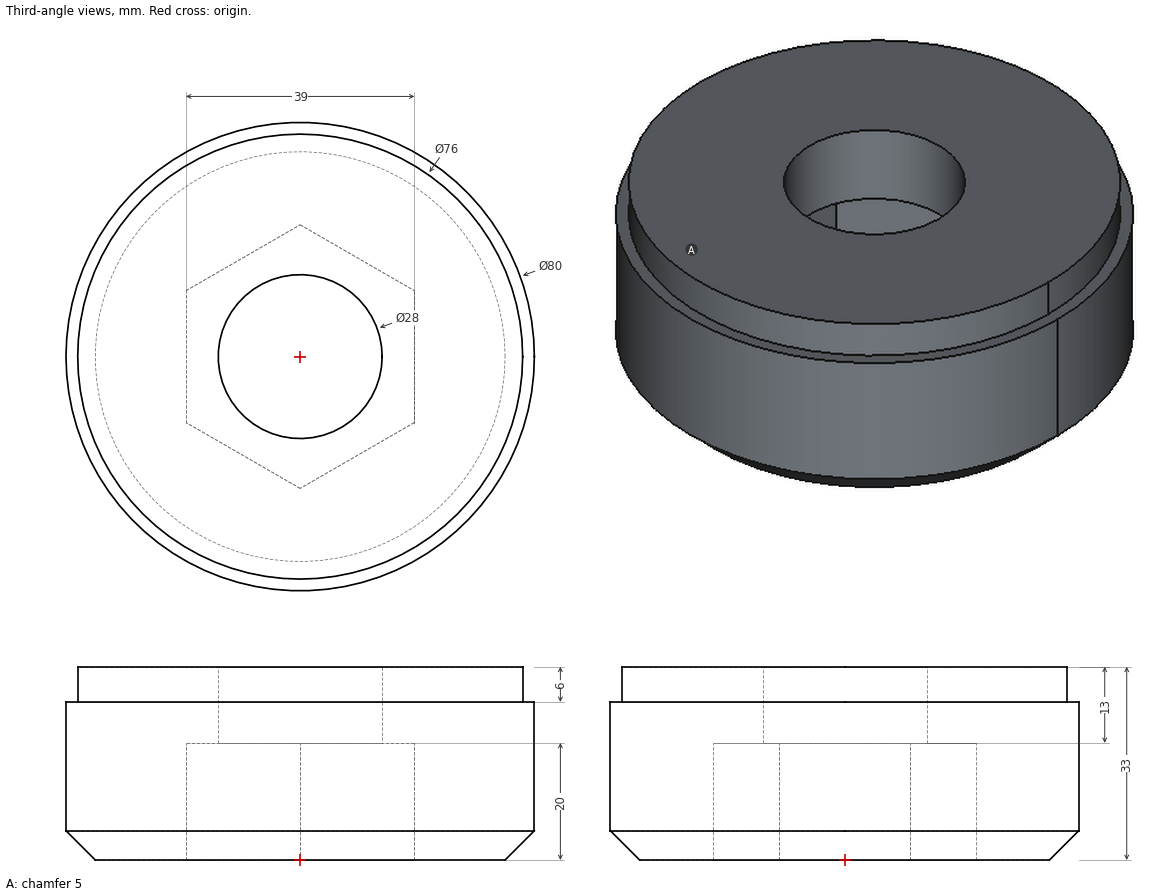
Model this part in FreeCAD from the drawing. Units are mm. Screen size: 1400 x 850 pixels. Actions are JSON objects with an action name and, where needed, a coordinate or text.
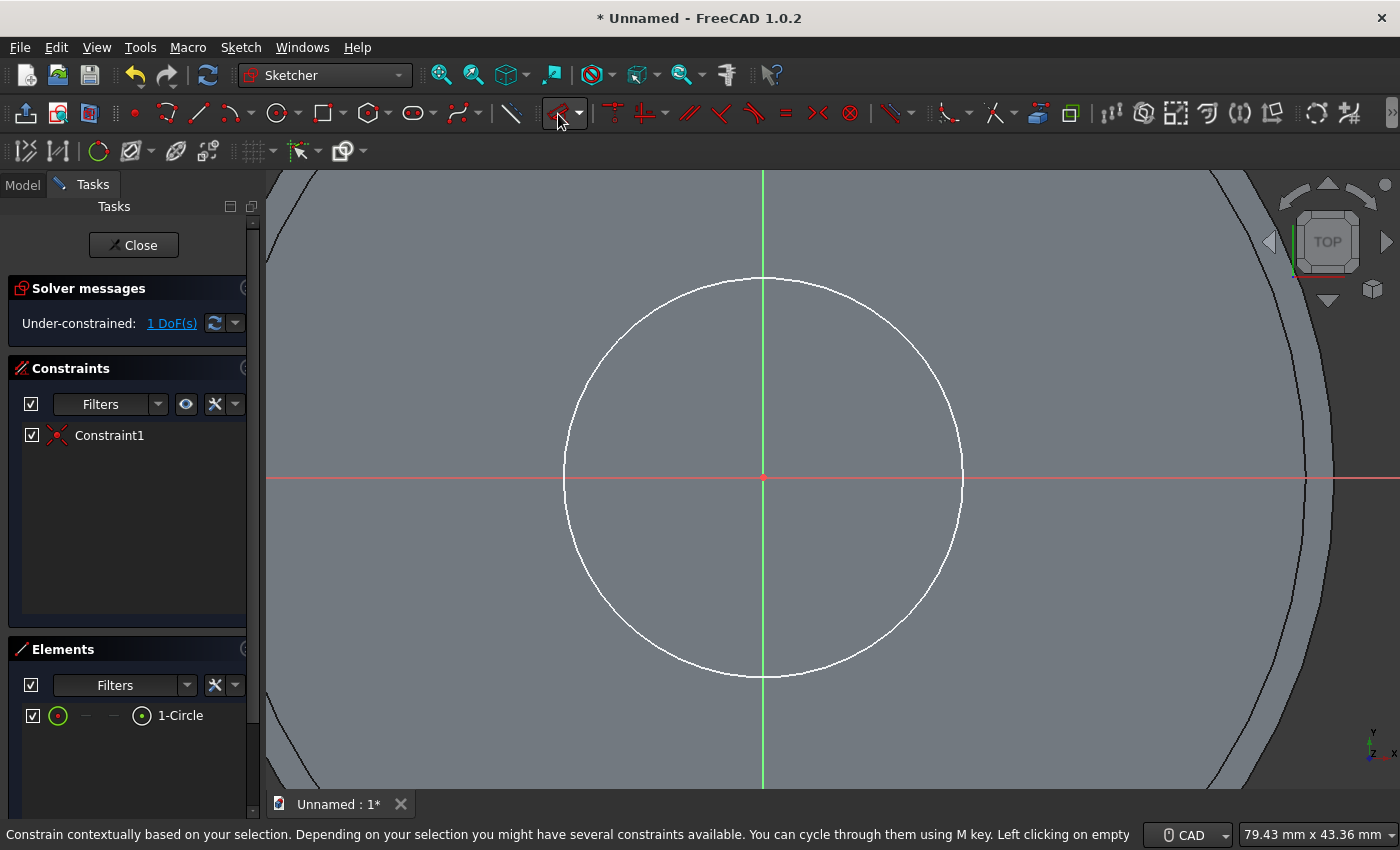
{"action": "left_click", "coordinate": [904, 336]}
{"action": "left_click", "coordinate": [927, 313]}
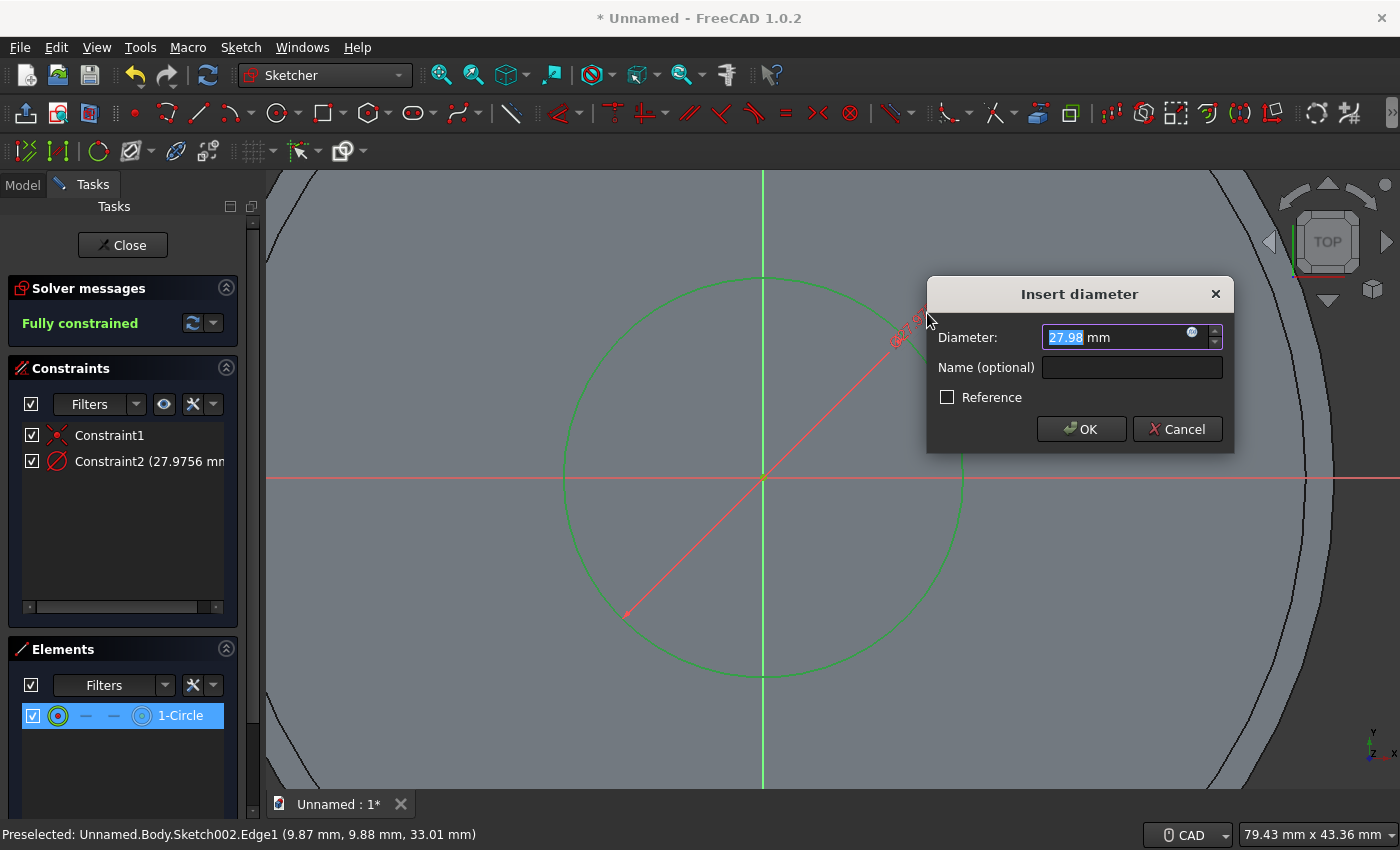
{"action": "type", "text": "28"}
{"action": "key", "text": "Return"}
{"action": "key", "text": "Escape"}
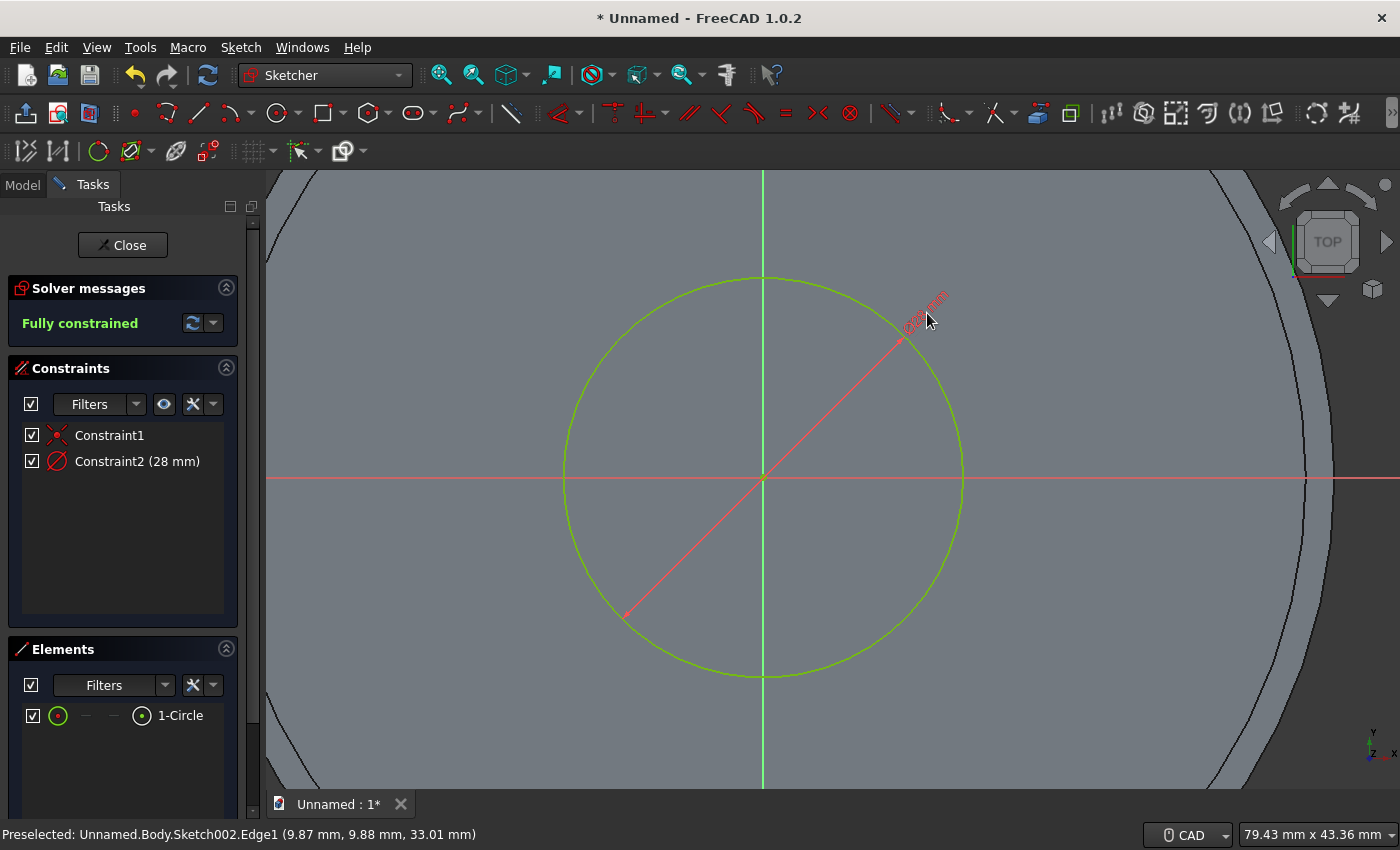
{"action": "left_click", "coordinate": [123, 245]}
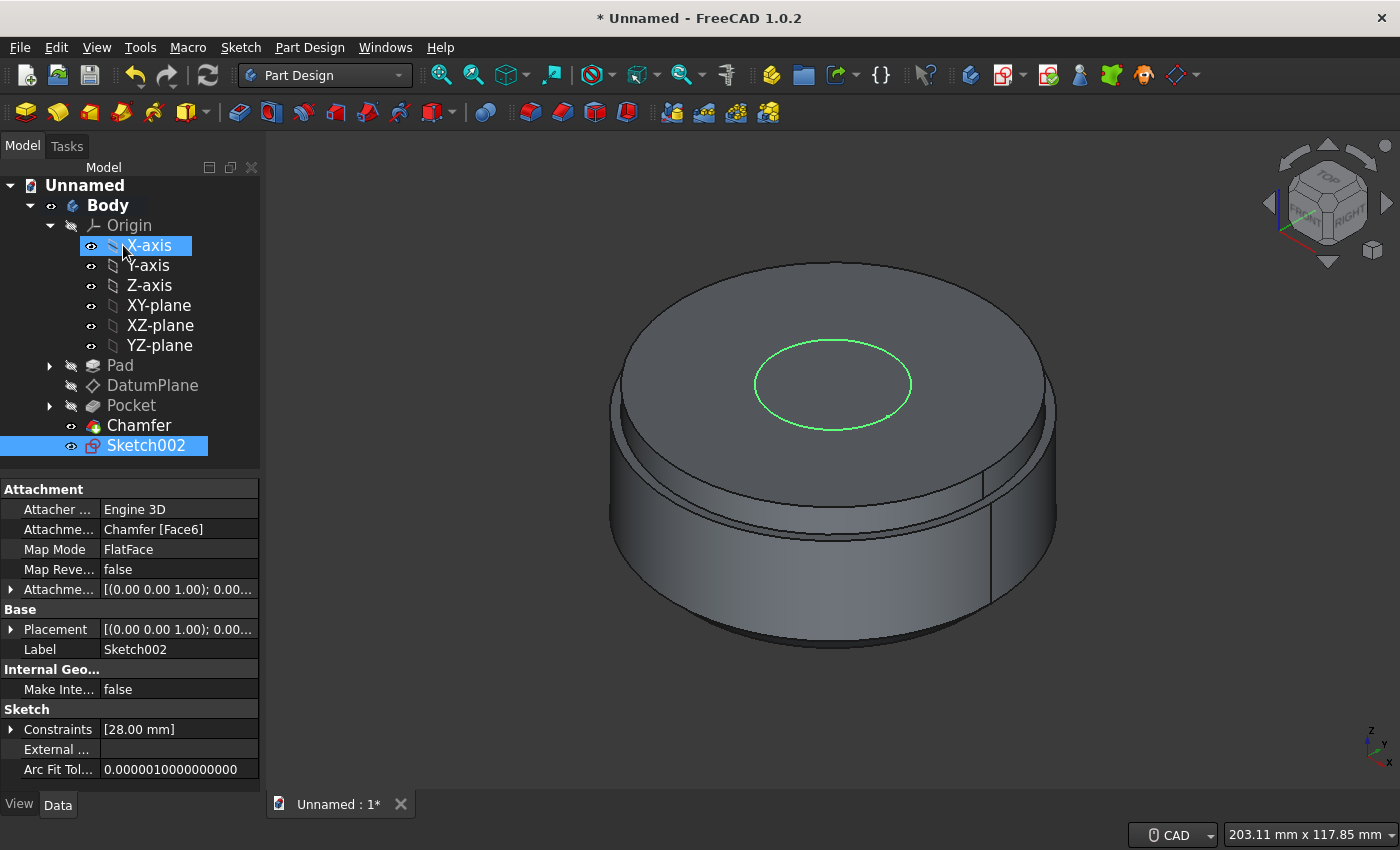
{"action": "left_click", "coordinate": [240, 112]}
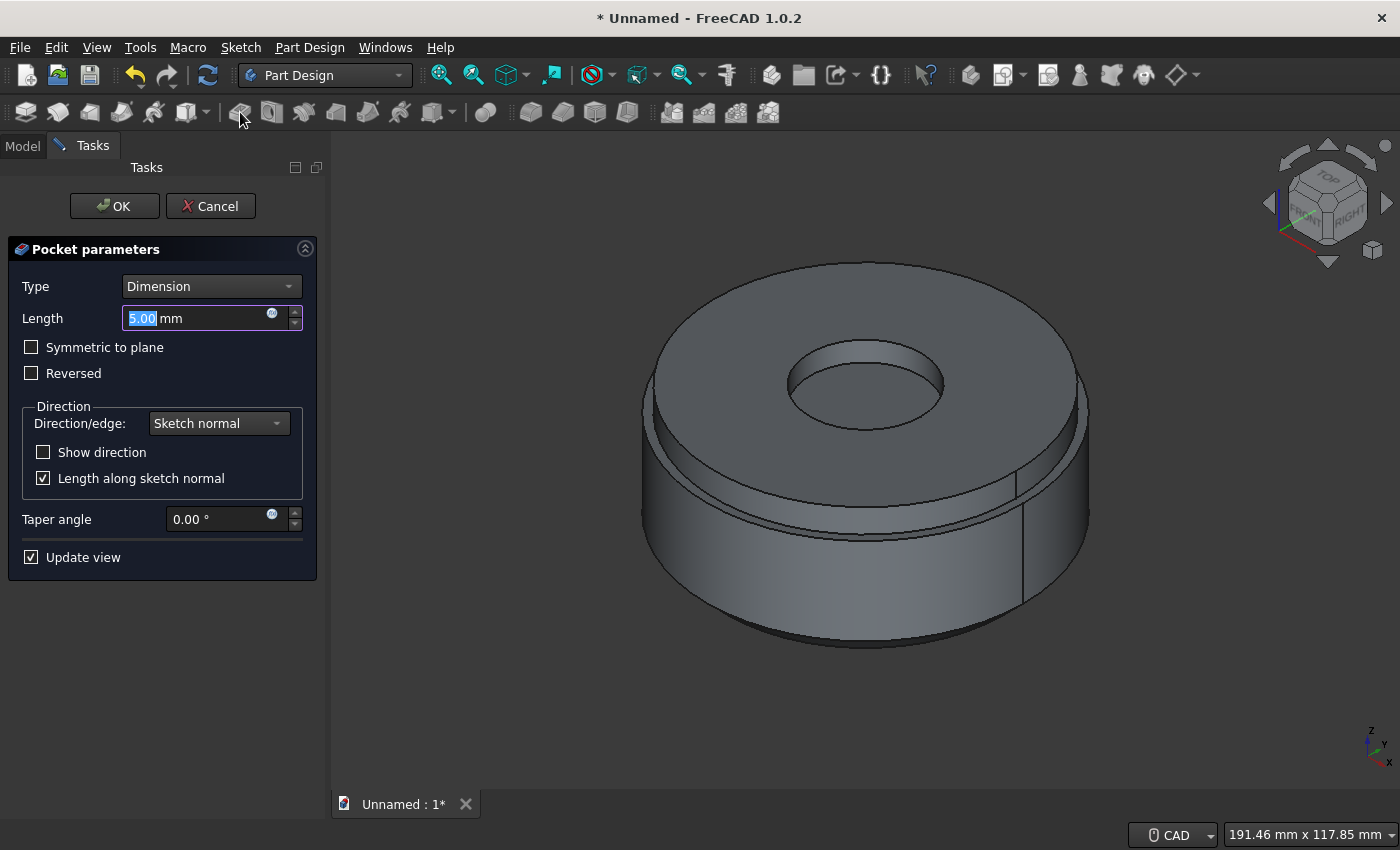
{"action": "type", "text": "13"}
{"action": "key", "text": "Tab"}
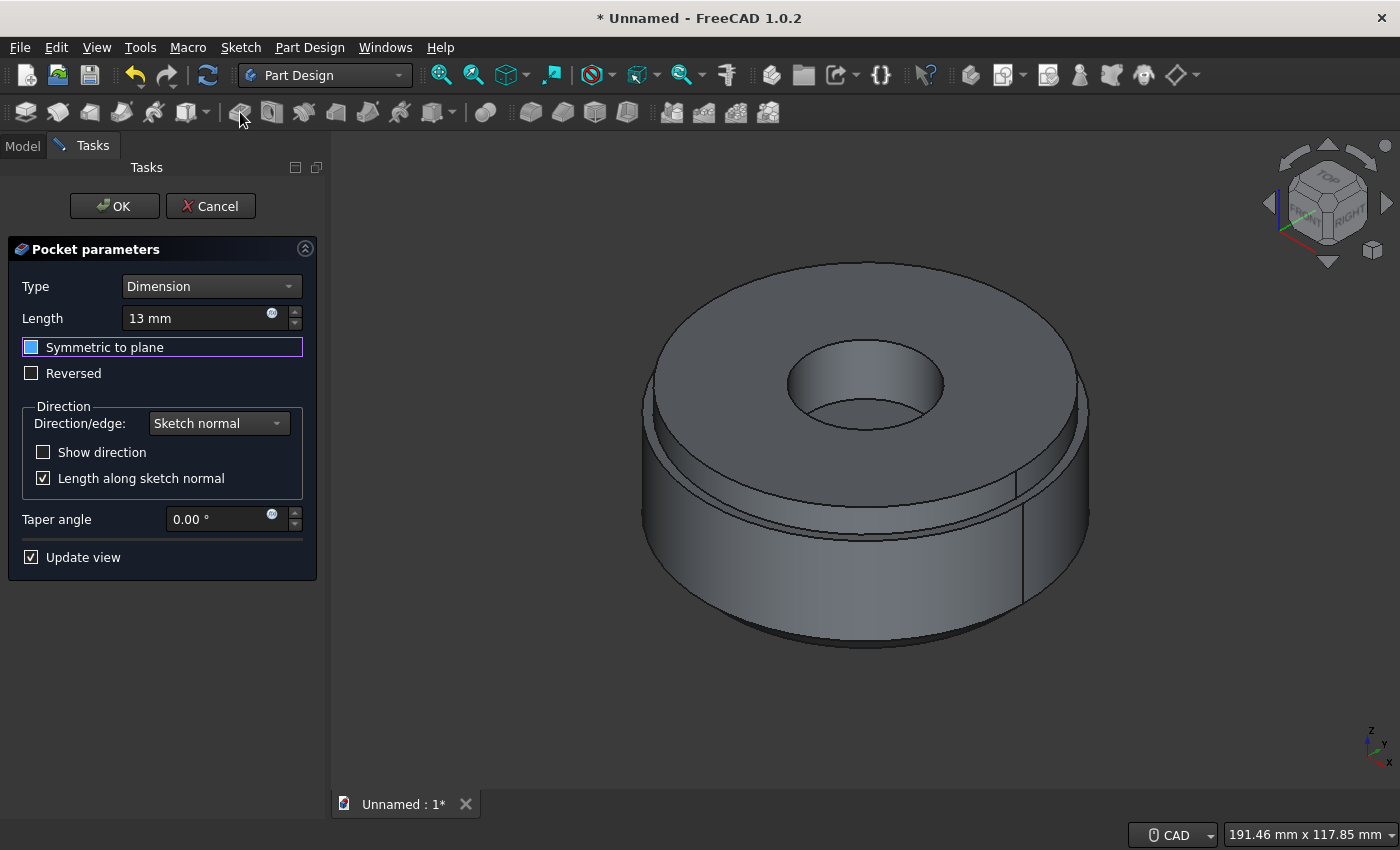
{"action": "left_click", "coordinate": [115, 206]}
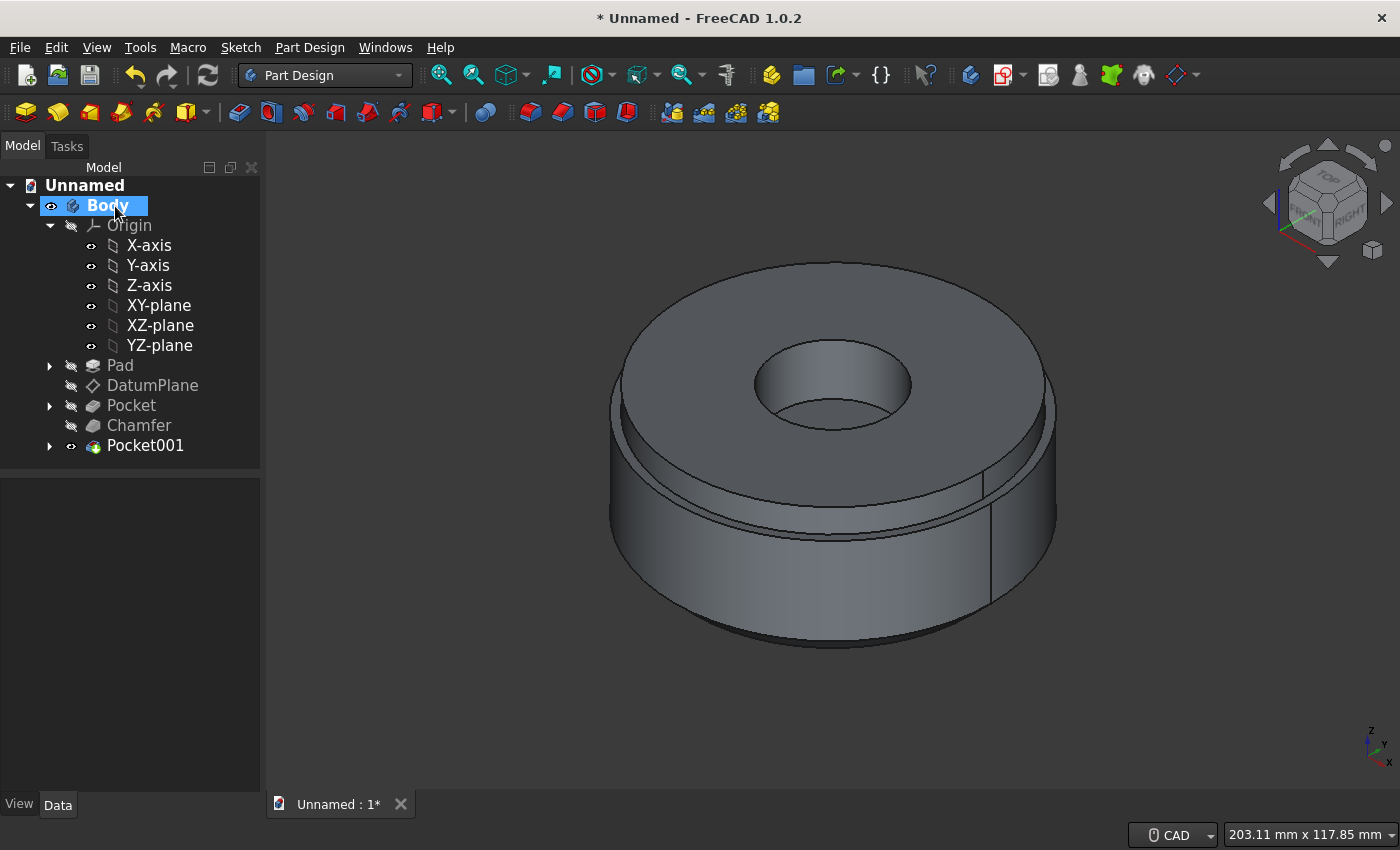
{"action": "left_click", "coordinate": [1004, 76]}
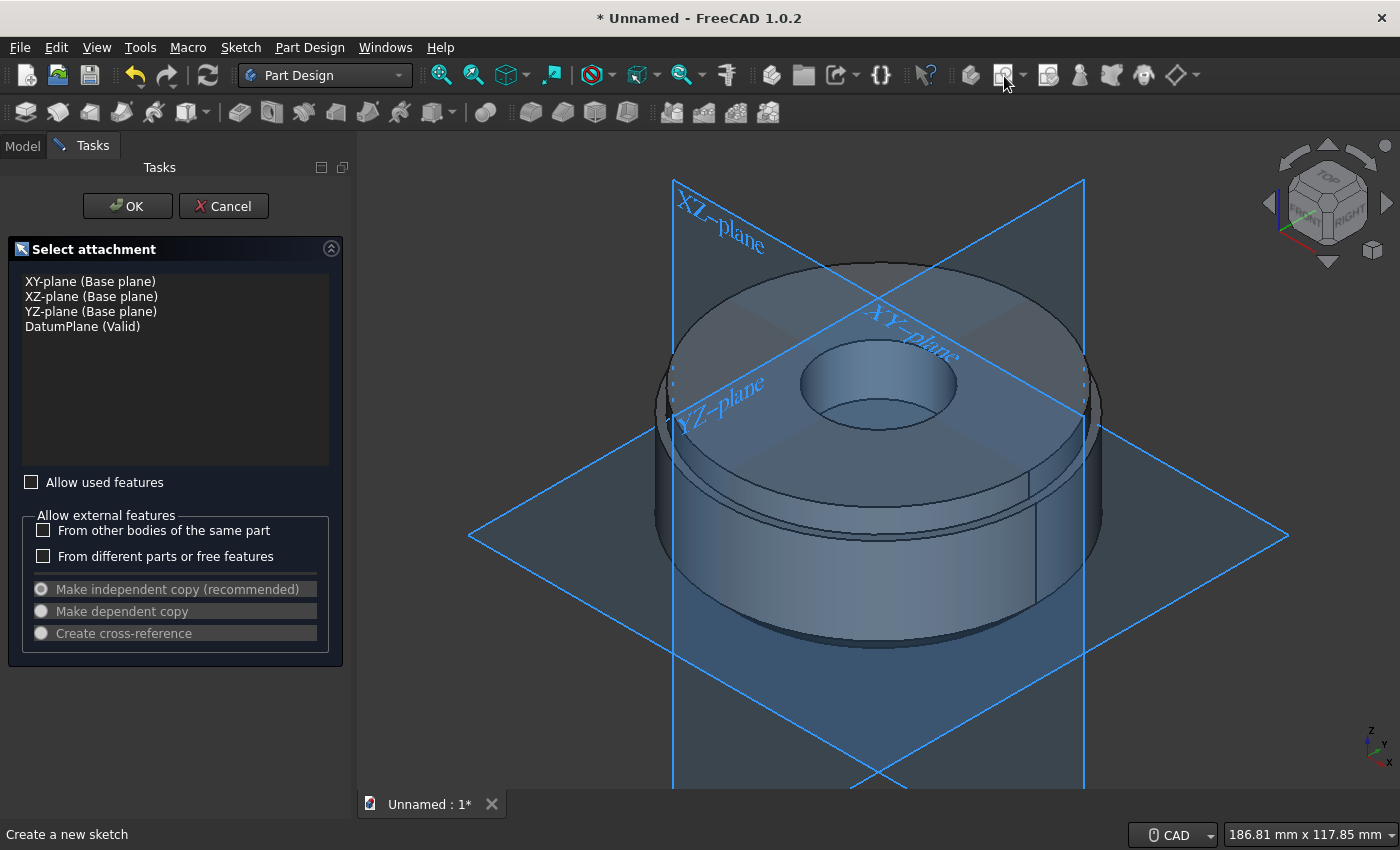
{"action": "left_click", "coordinate": [82, 282]}